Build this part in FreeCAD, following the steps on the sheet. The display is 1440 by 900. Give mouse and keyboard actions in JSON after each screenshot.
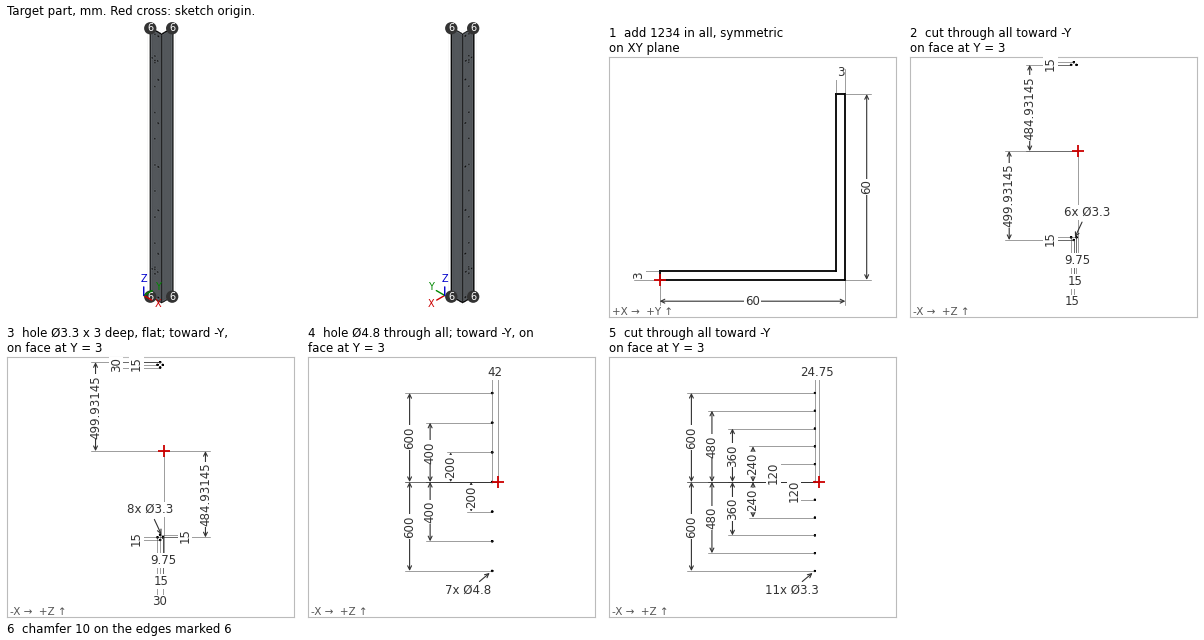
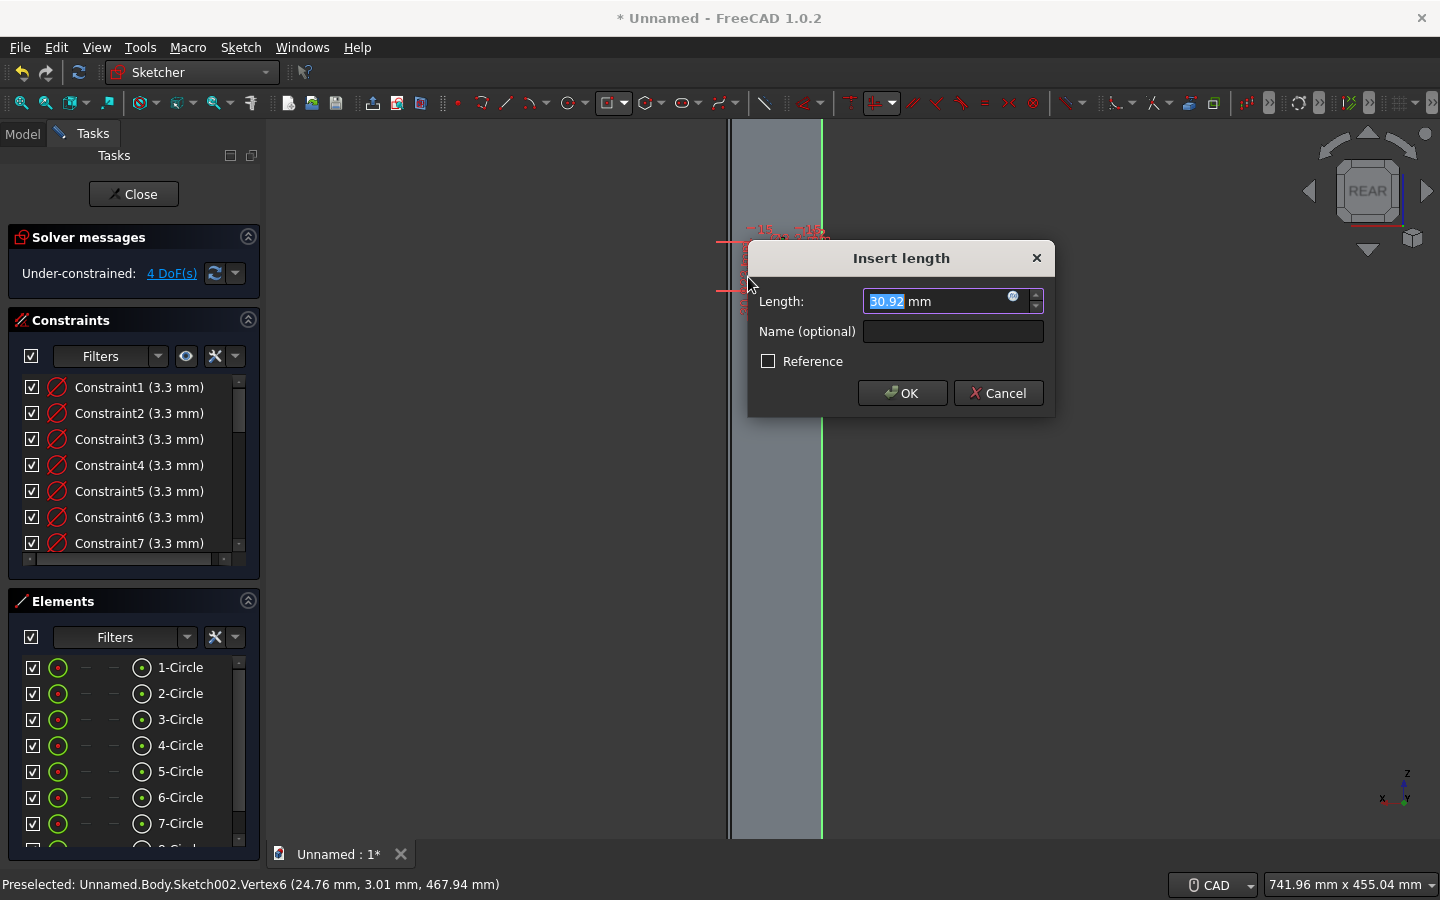
{"action": "type", "text": "30"}
{"action": "key", "text": "Return"}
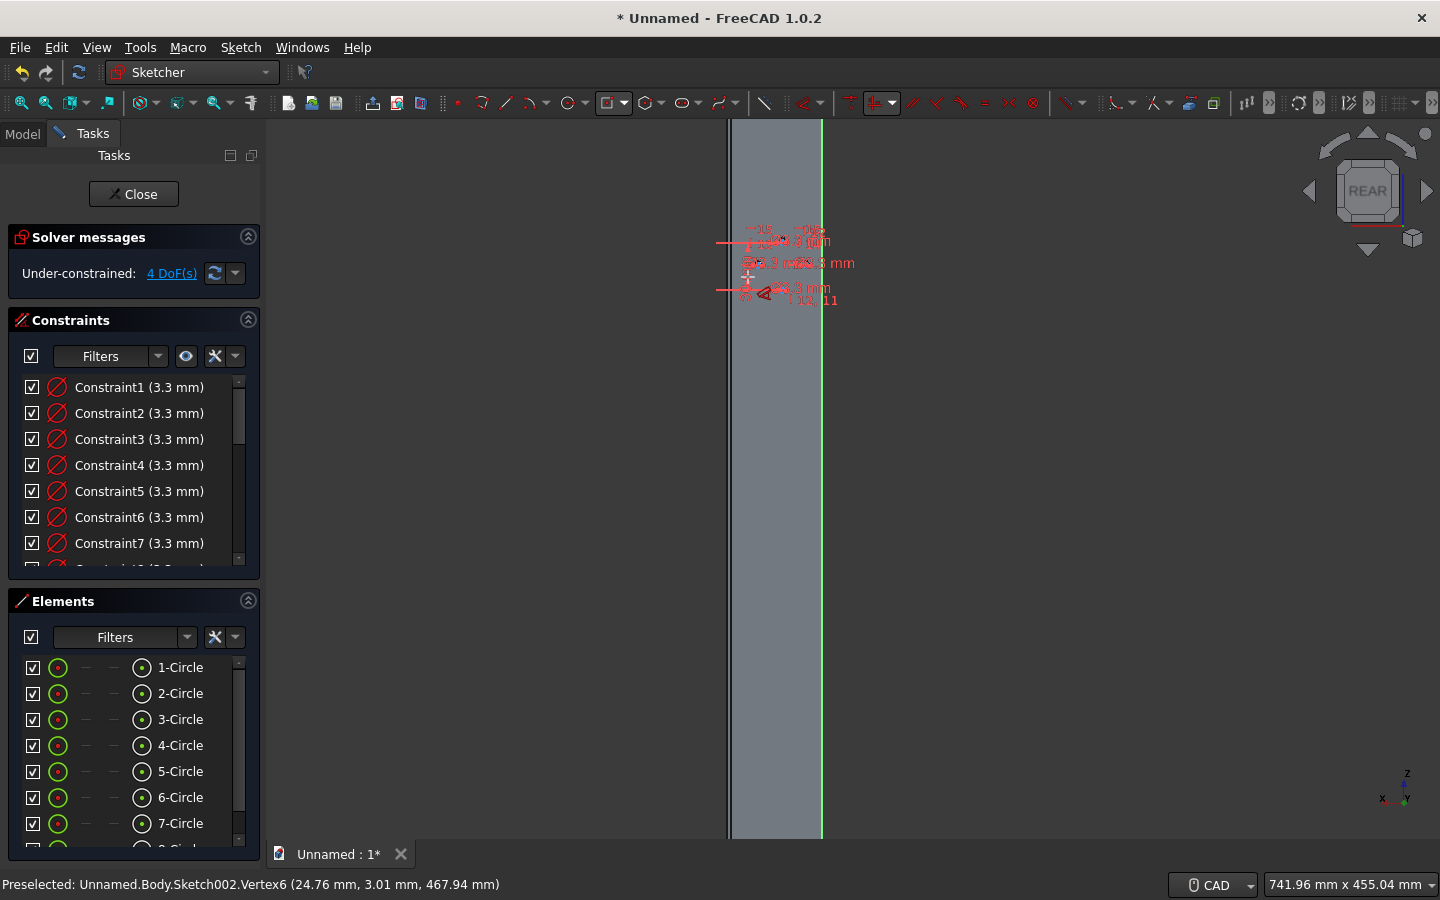
{"action": "scroll", "coordinate": [782, 243], "scroll_direction": "up", "scroll_amount": 3}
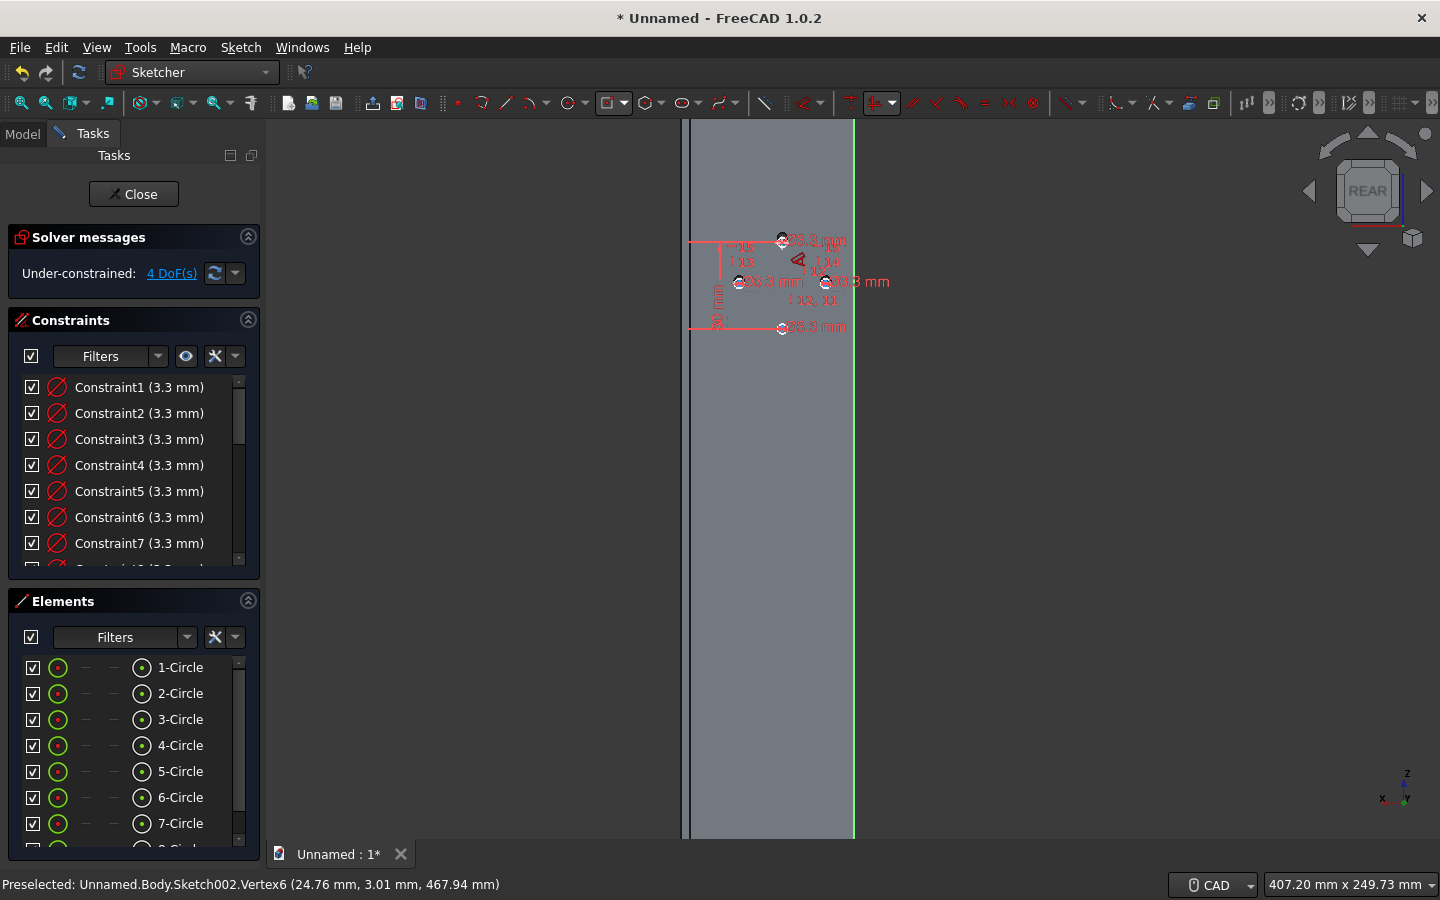
{"action": "left_click", "coordinate": [783, 242]}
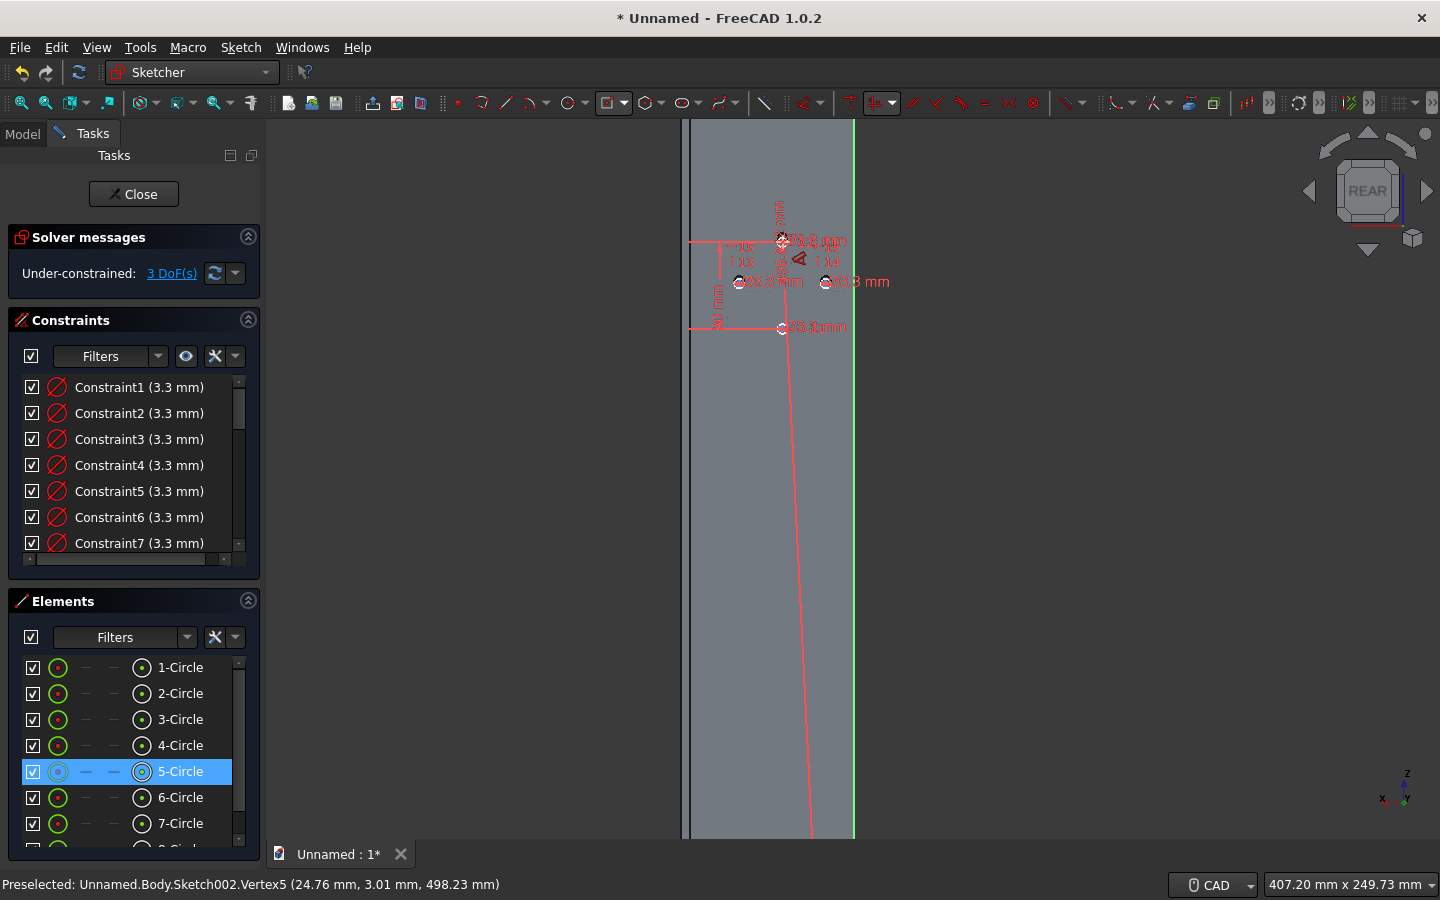
{"action": "left_click", "coordinate": [739, 284]}
{"action": "left_click", "coordinate": [705, 263]}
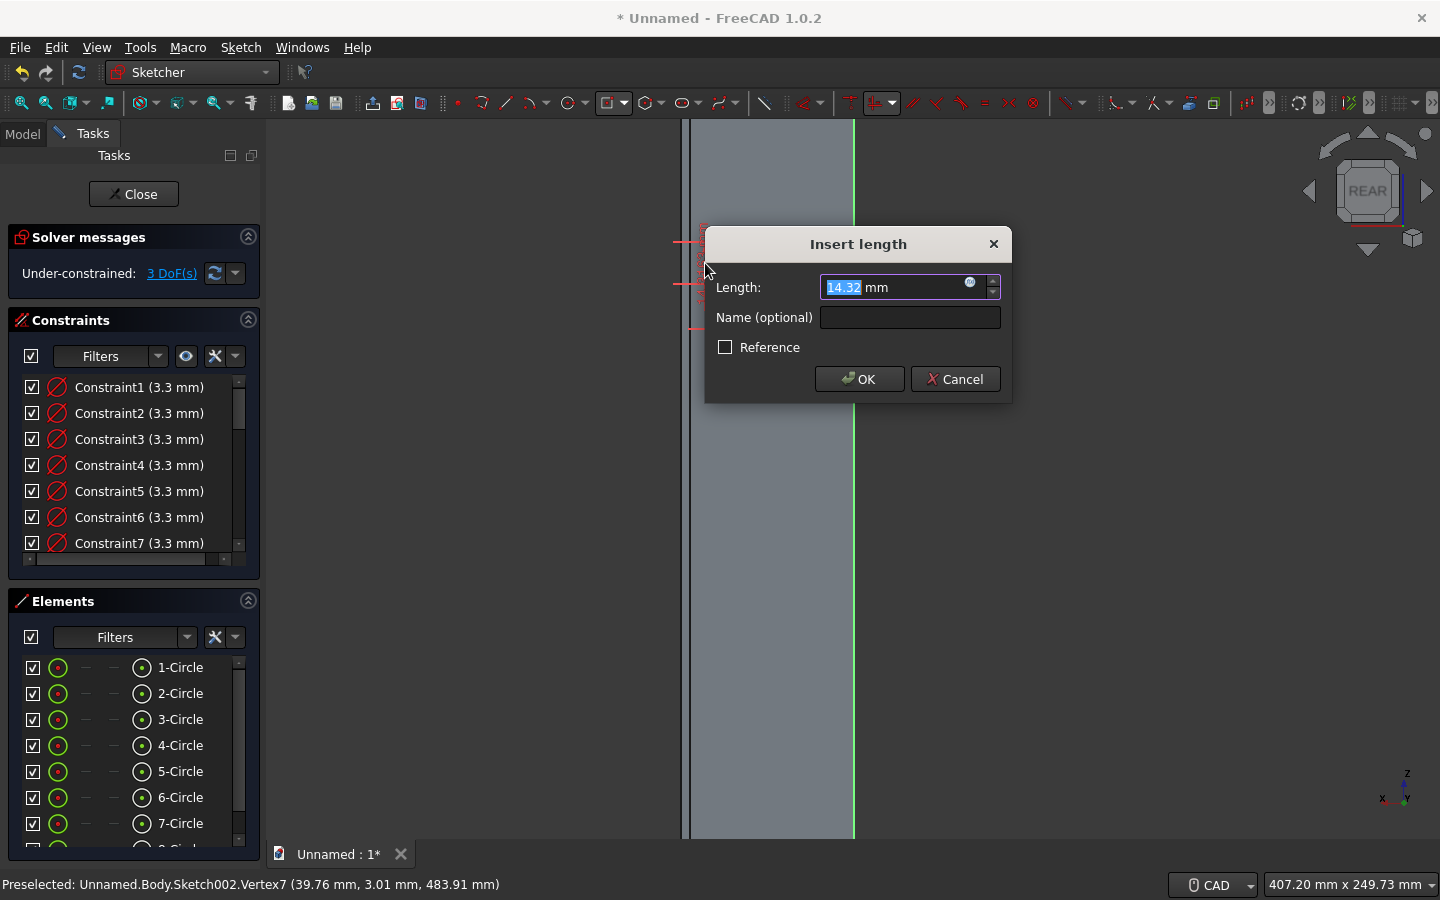
{"action": "type", "text": "15"}
{"action": "key", "text": "Return"}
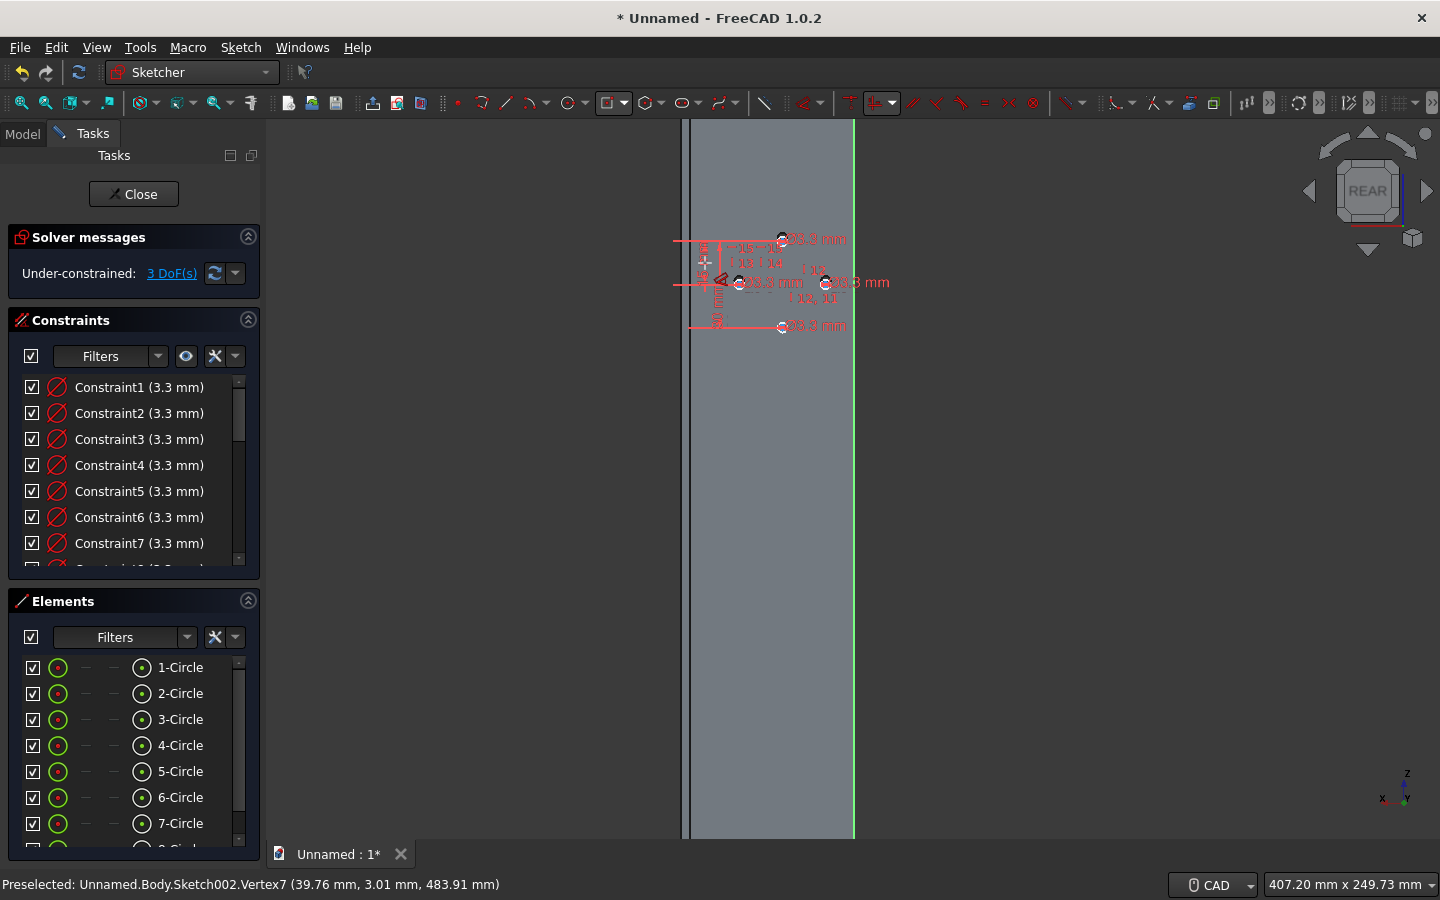
{"action": "scroll", "coordinate": [783, 241], "scroll_direction": "down", "scroll_amount": 9}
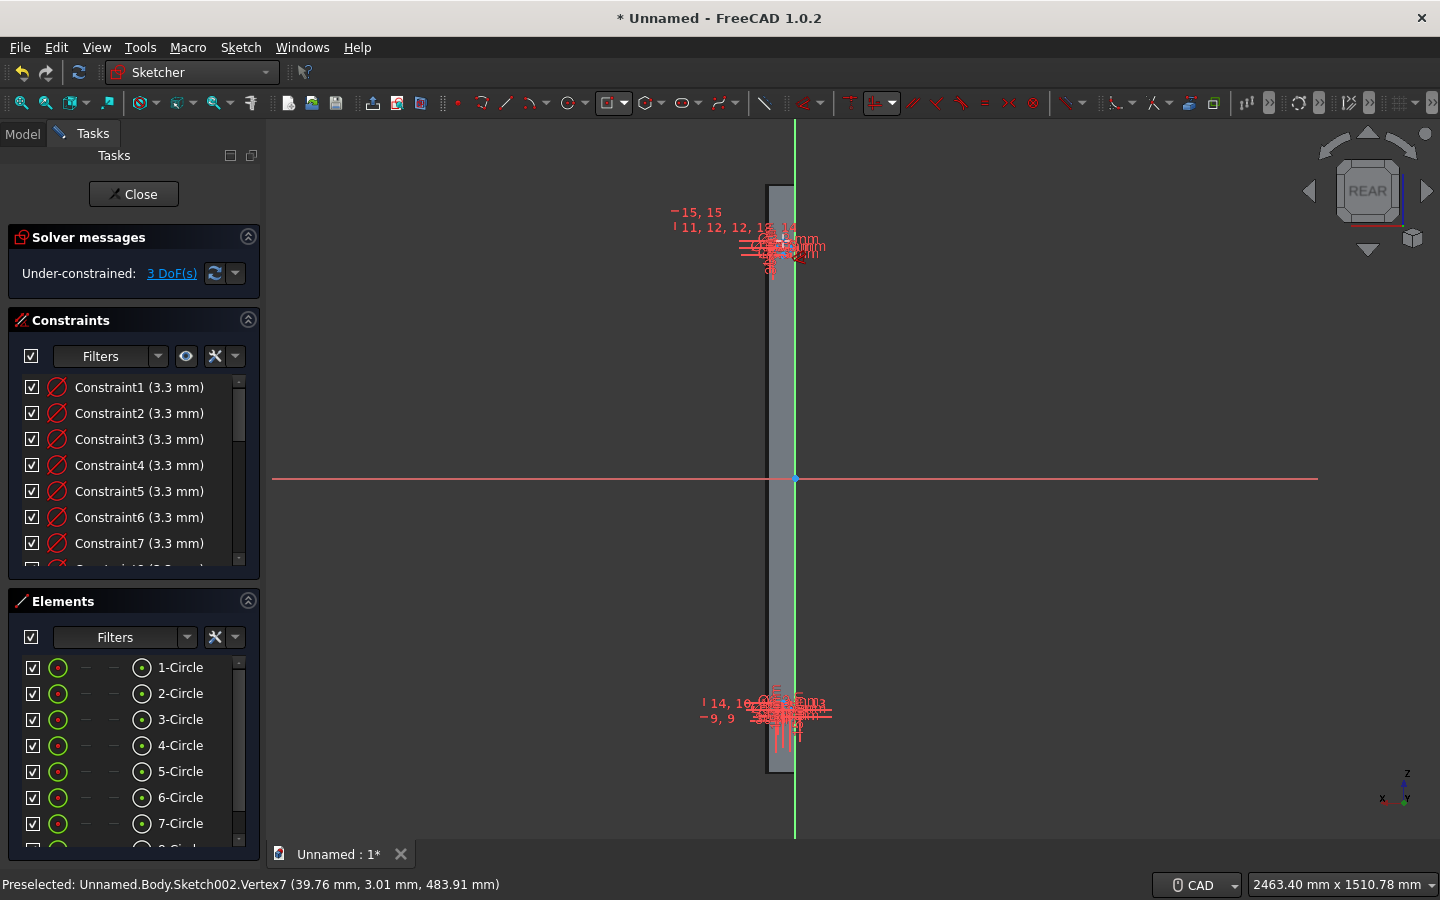
{"action": "scroll", "coordinate": [790, 710], "scroll_direction": "up", "scroll_amount": 11}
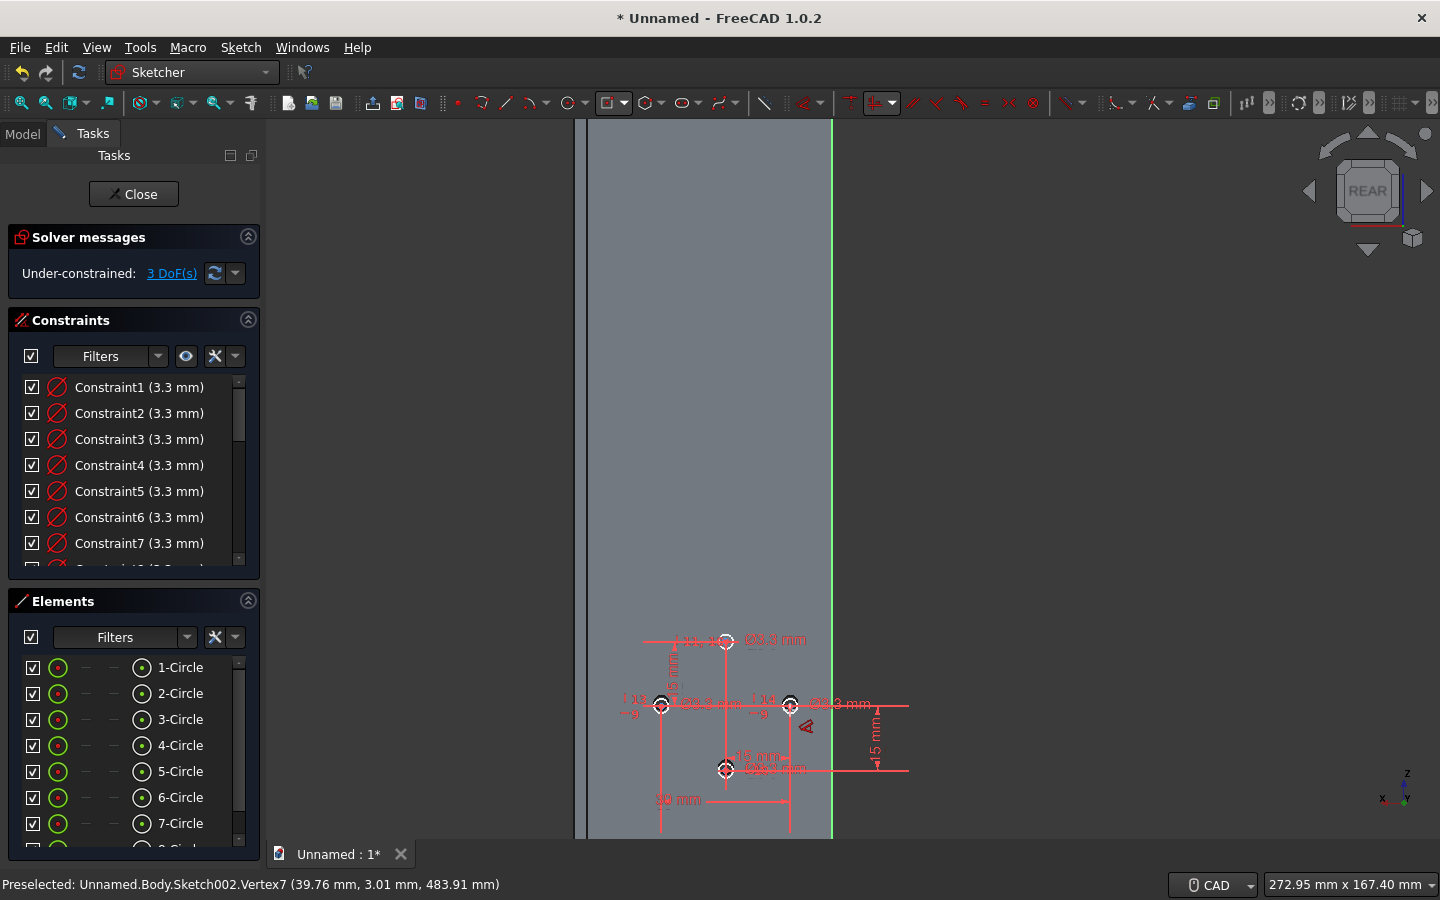
{"action": "left_click", "coordinate": [790, 706]}
{"action": "left_click", "coordinate": [811, 788]}